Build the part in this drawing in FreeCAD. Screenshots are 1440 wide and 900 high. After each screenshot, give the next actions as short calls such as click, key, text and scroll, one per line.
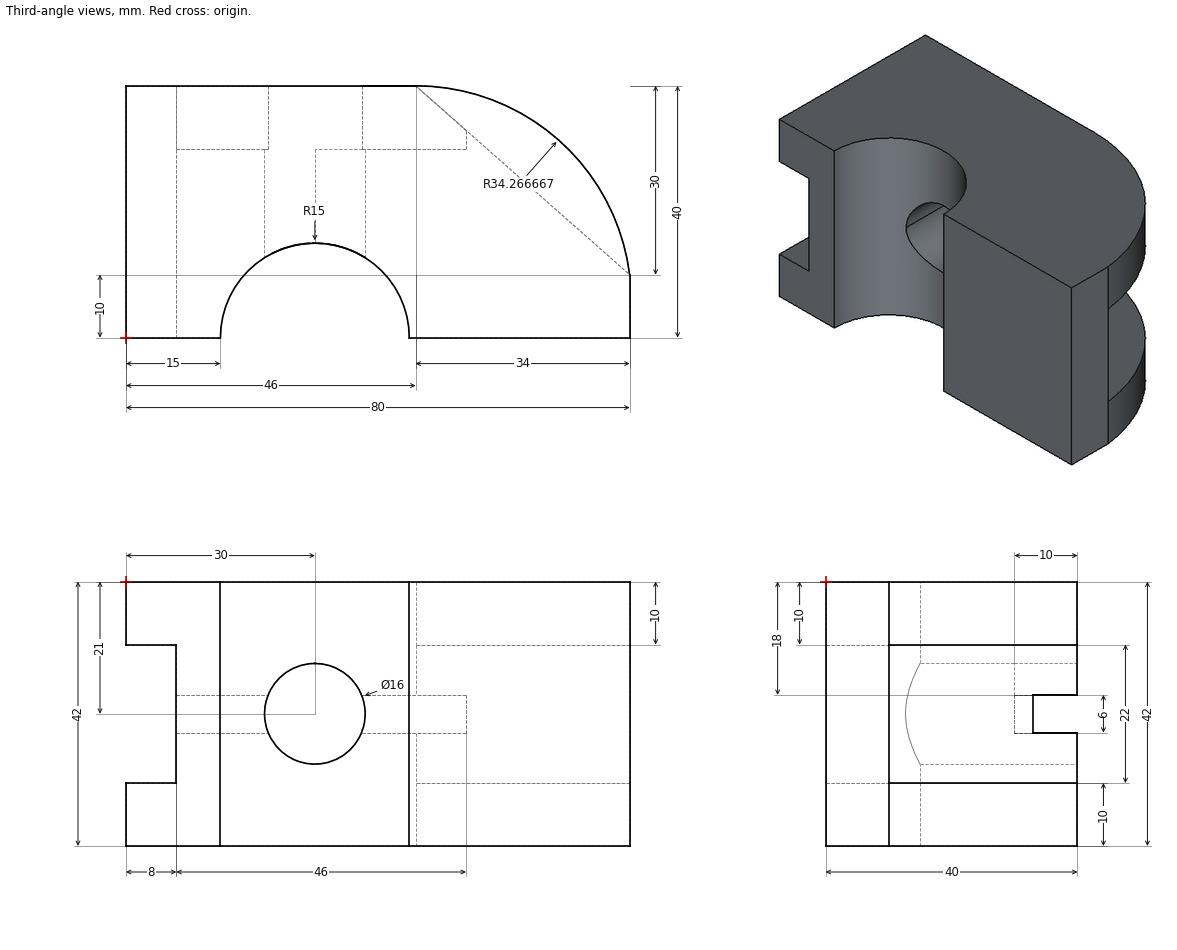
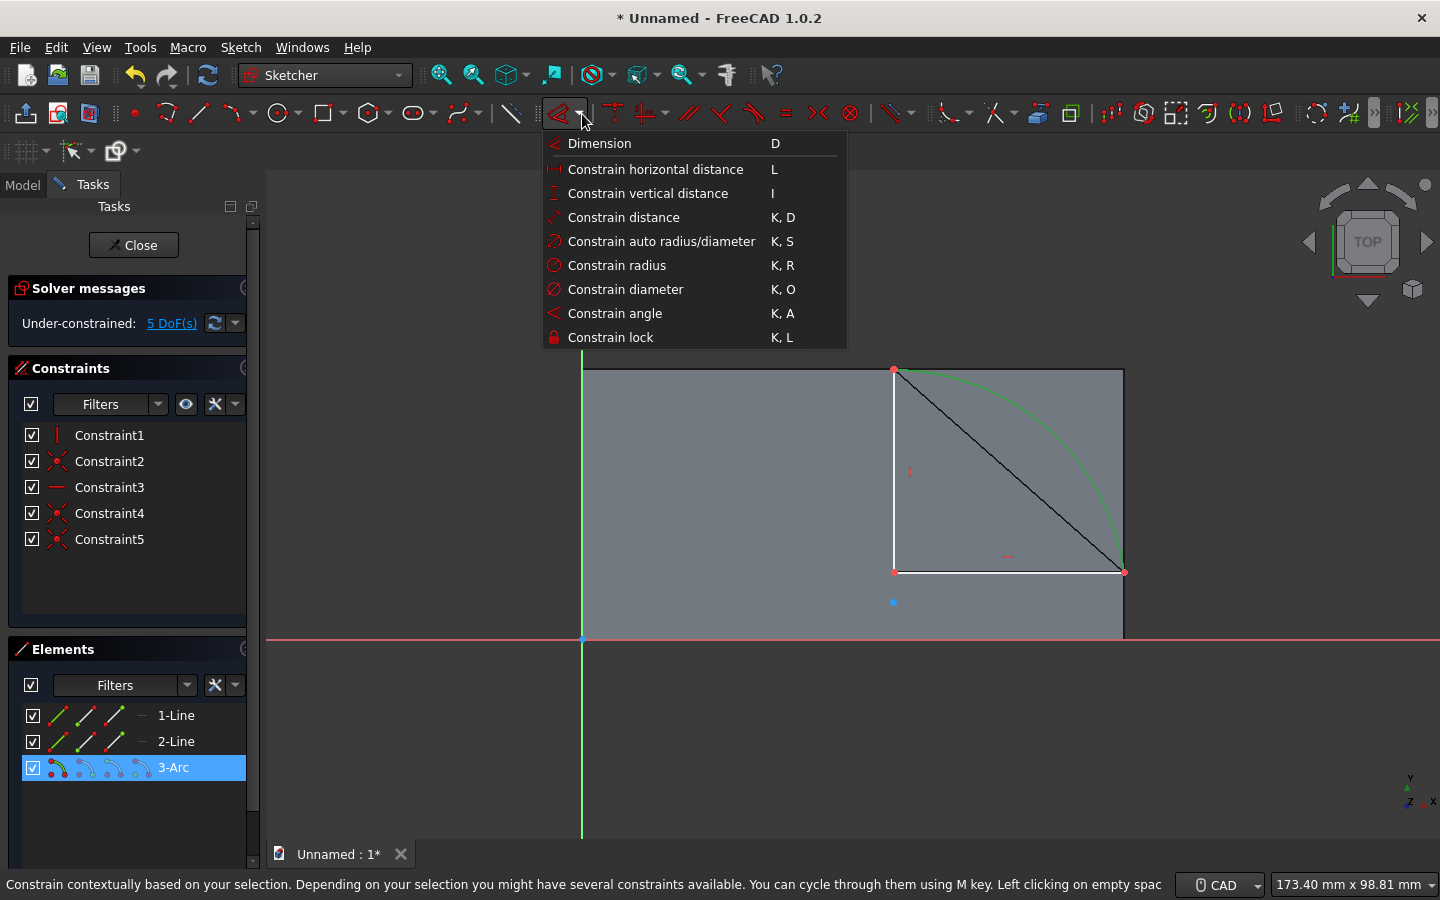
click(695, 265)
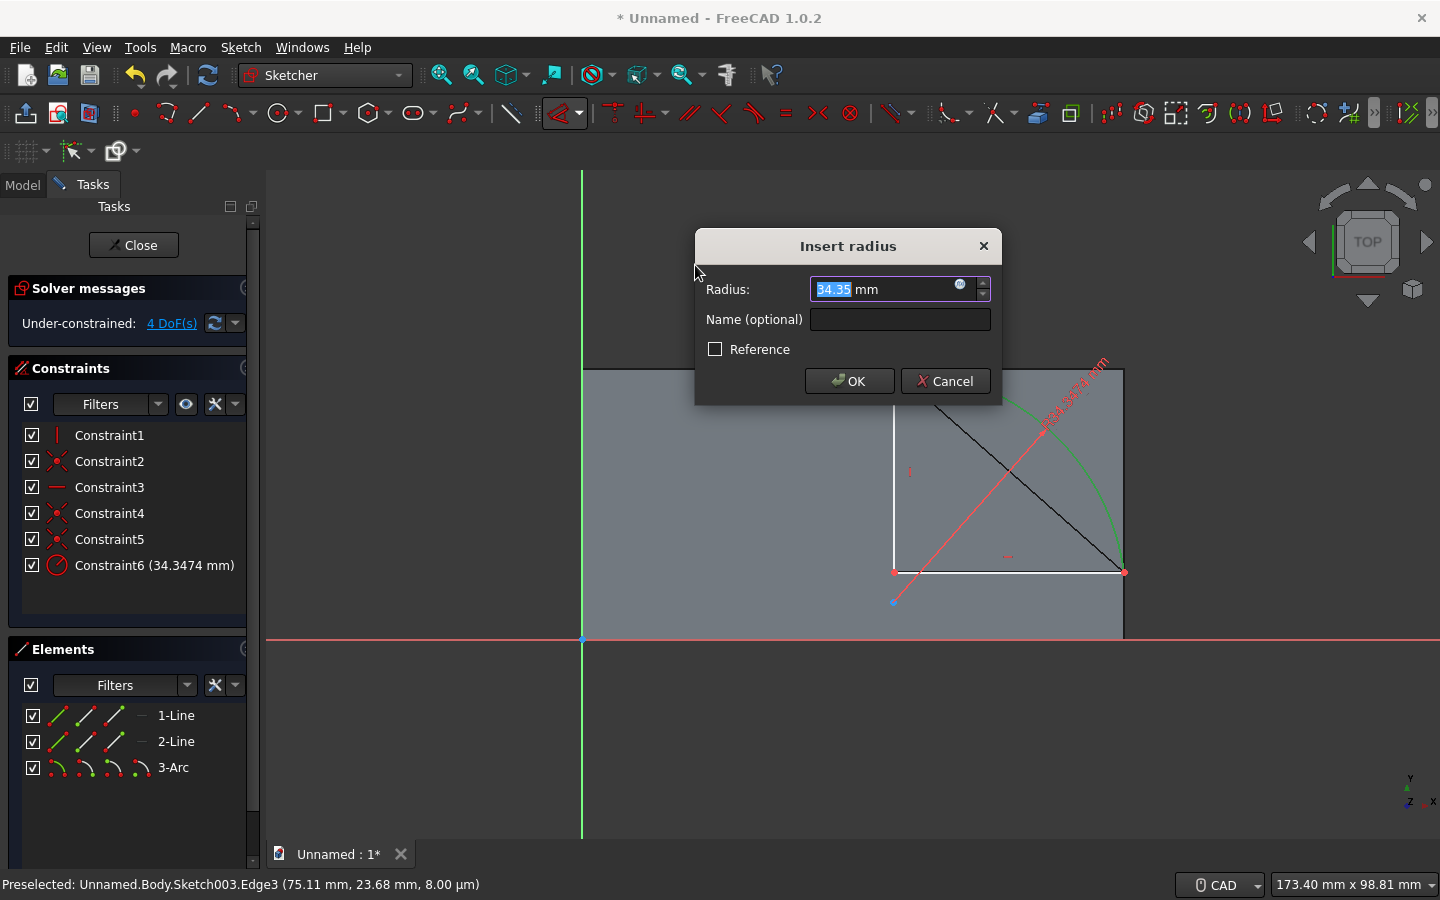
text(34.266667)
key(Return)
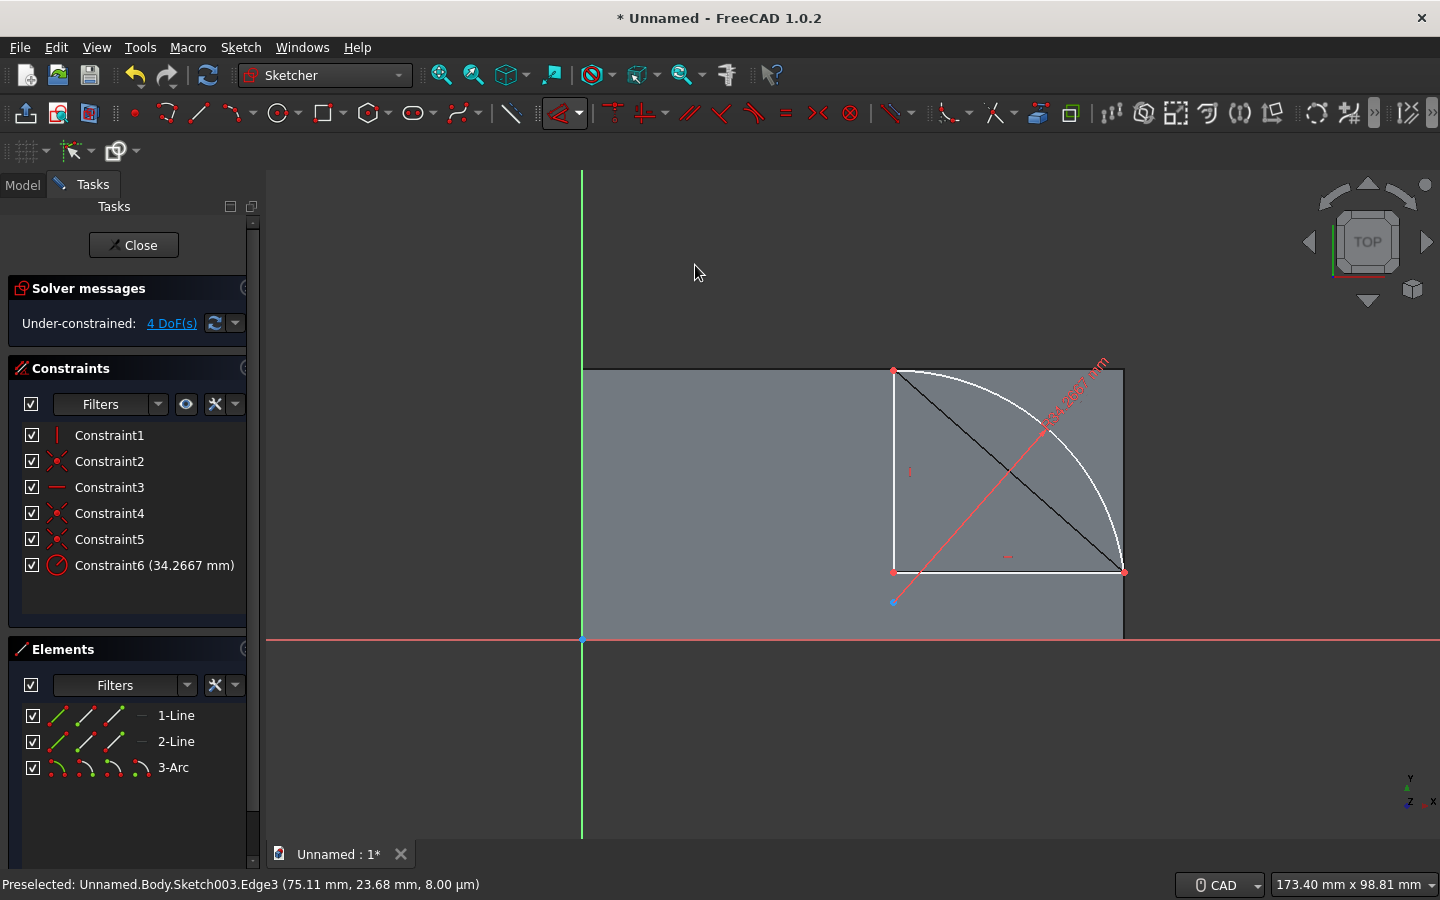
click(894, 431)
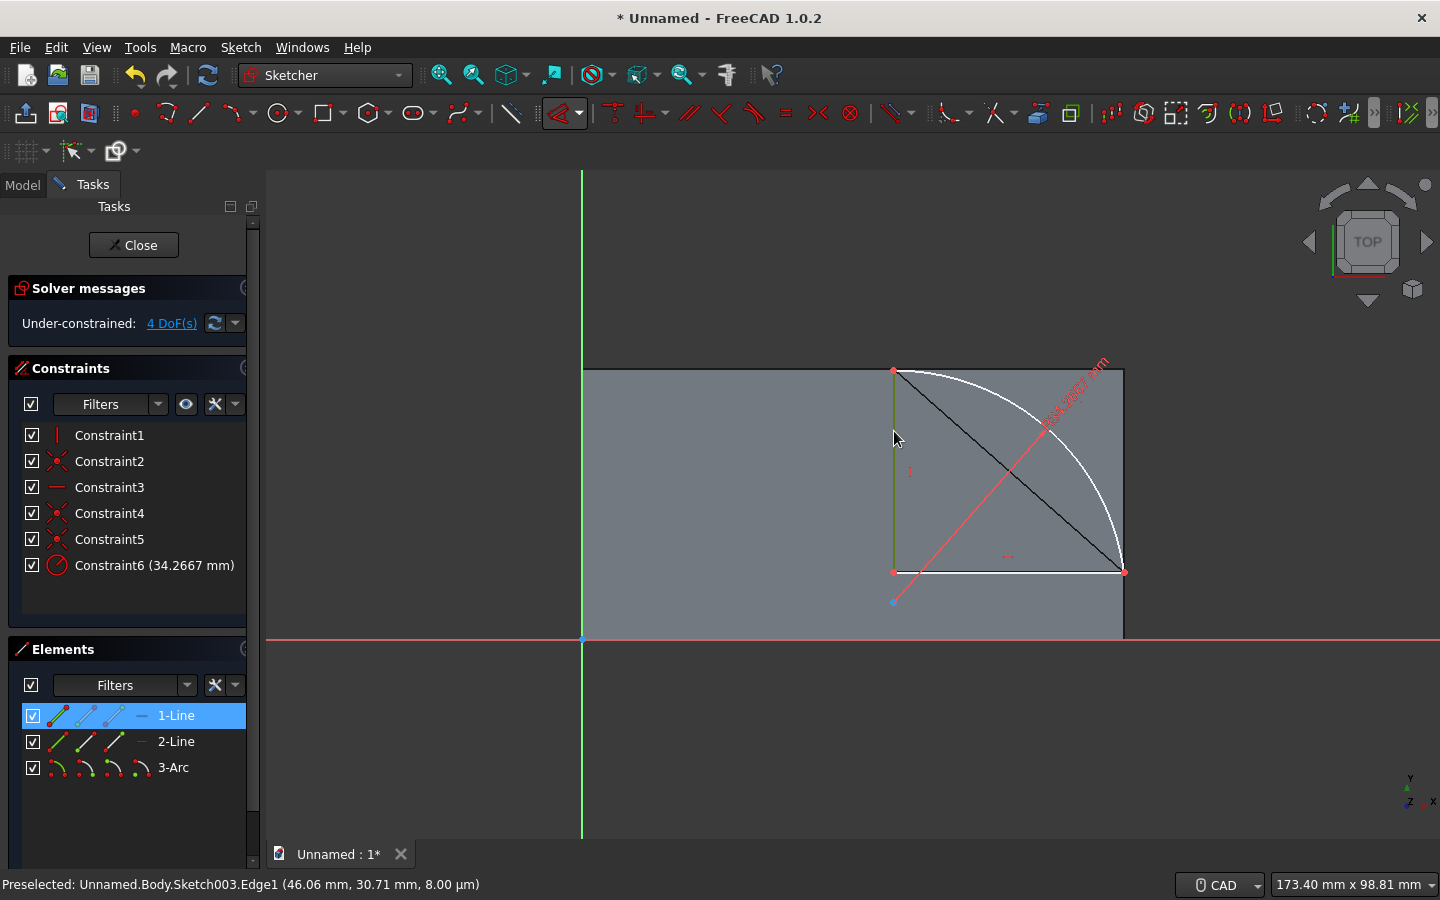
key(i)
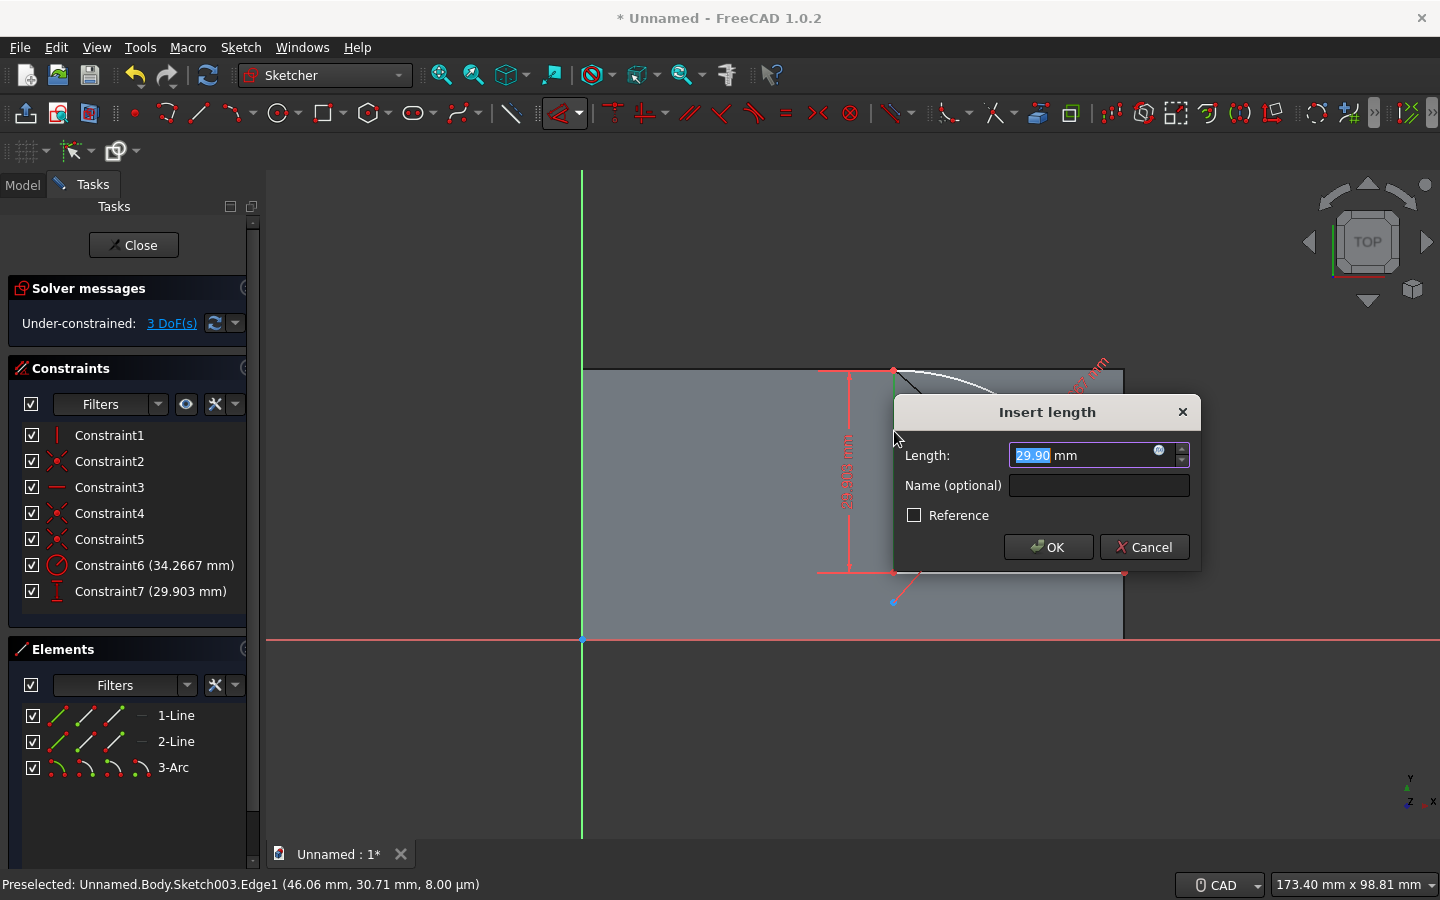
text(30)
key(Return)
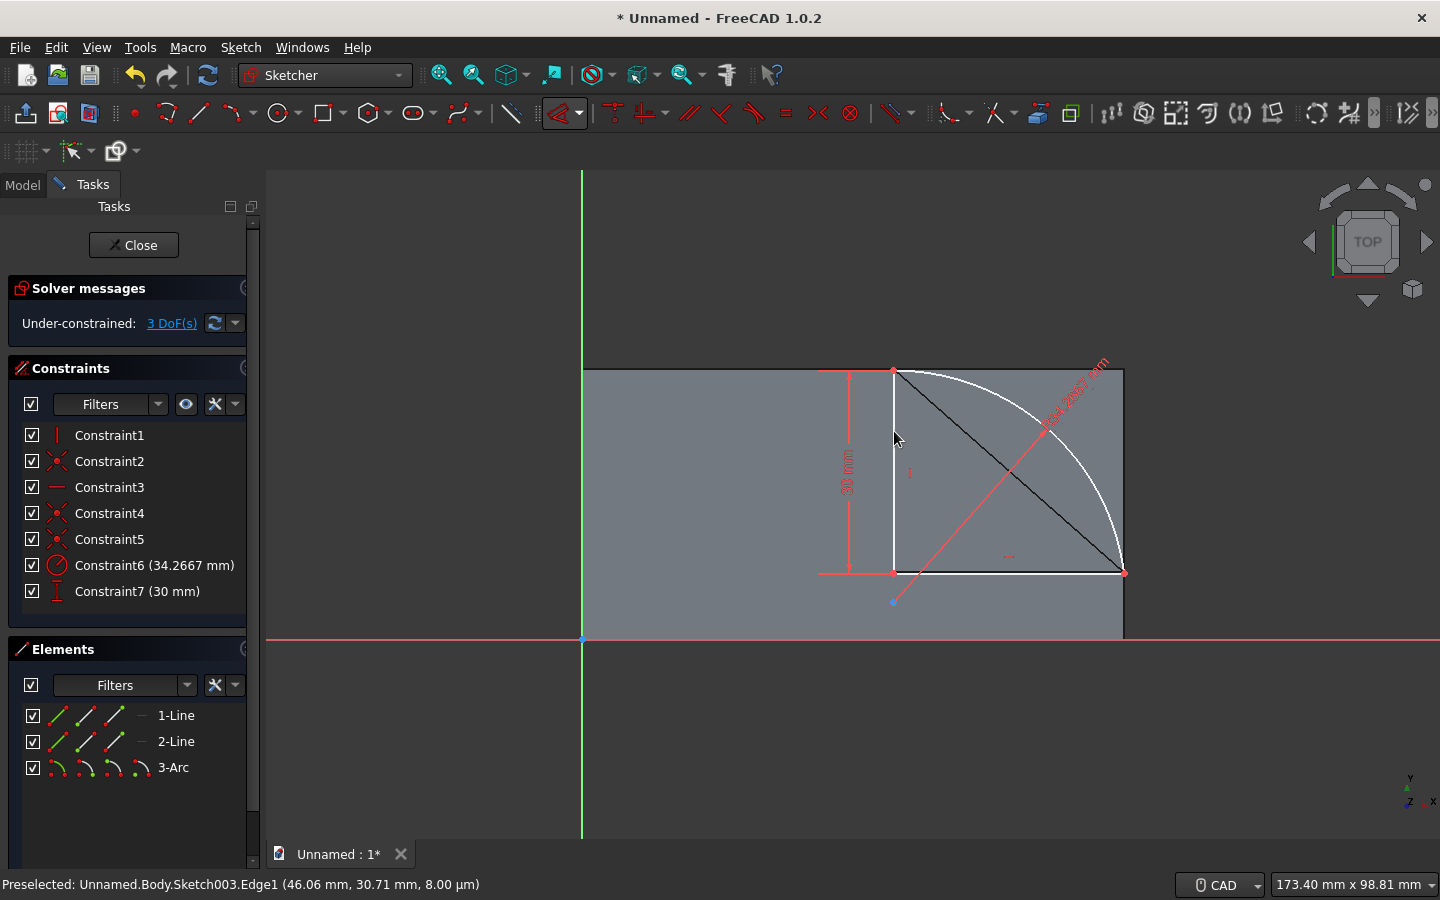
click(963, 574)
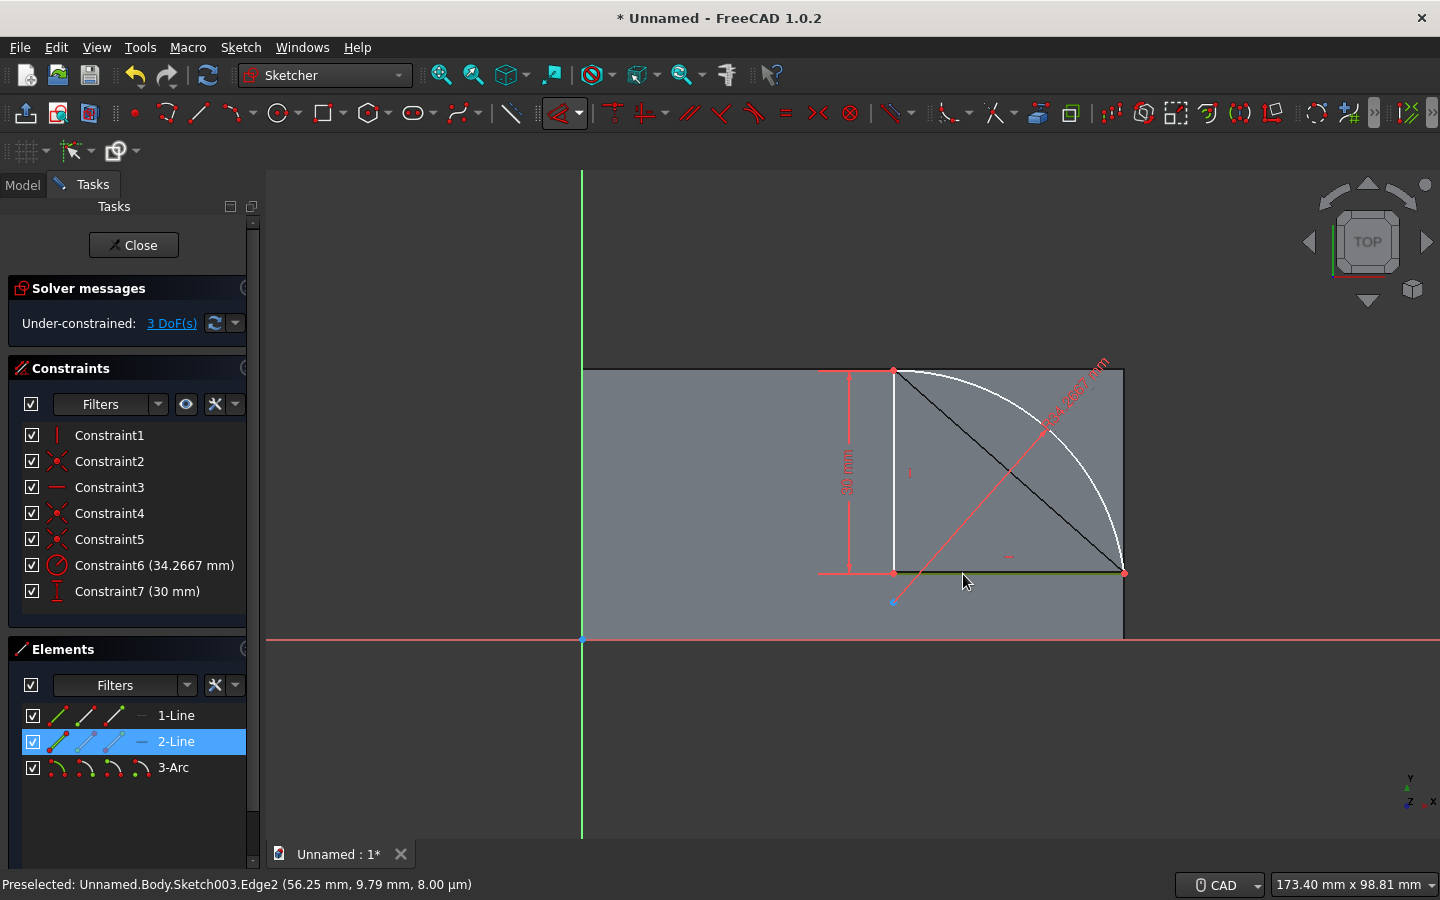
click(582, 114)